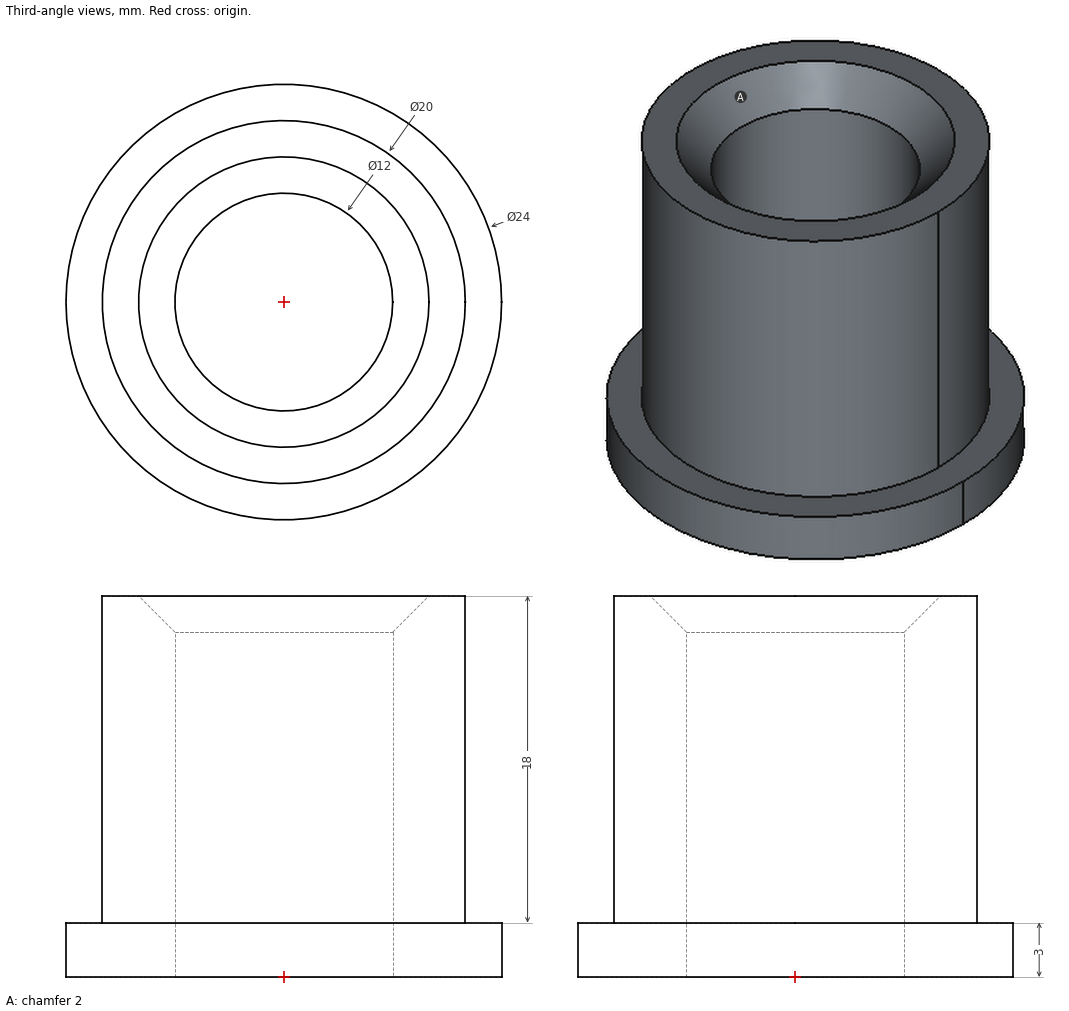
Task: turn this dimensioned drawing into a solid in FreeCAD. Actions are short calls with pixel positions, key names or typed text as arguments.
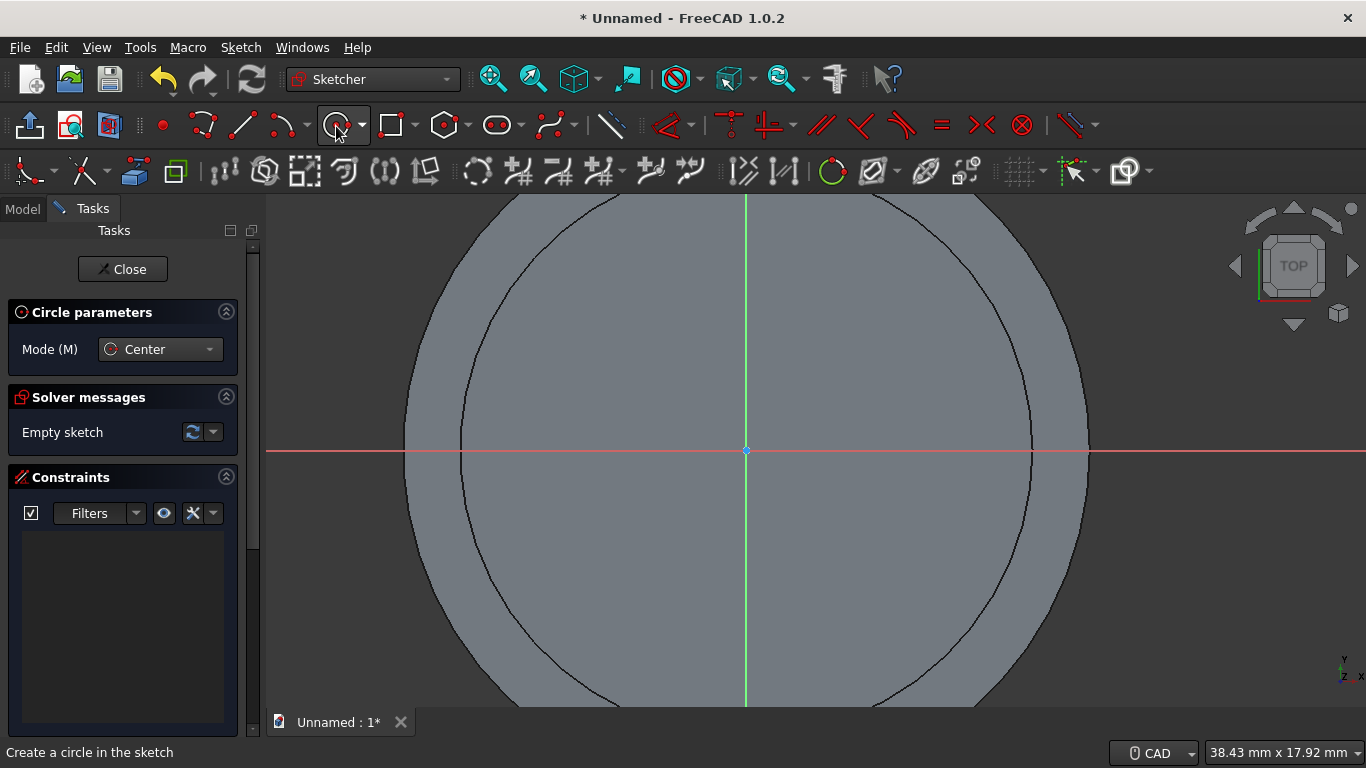
click(746, 450)
move(868, 329)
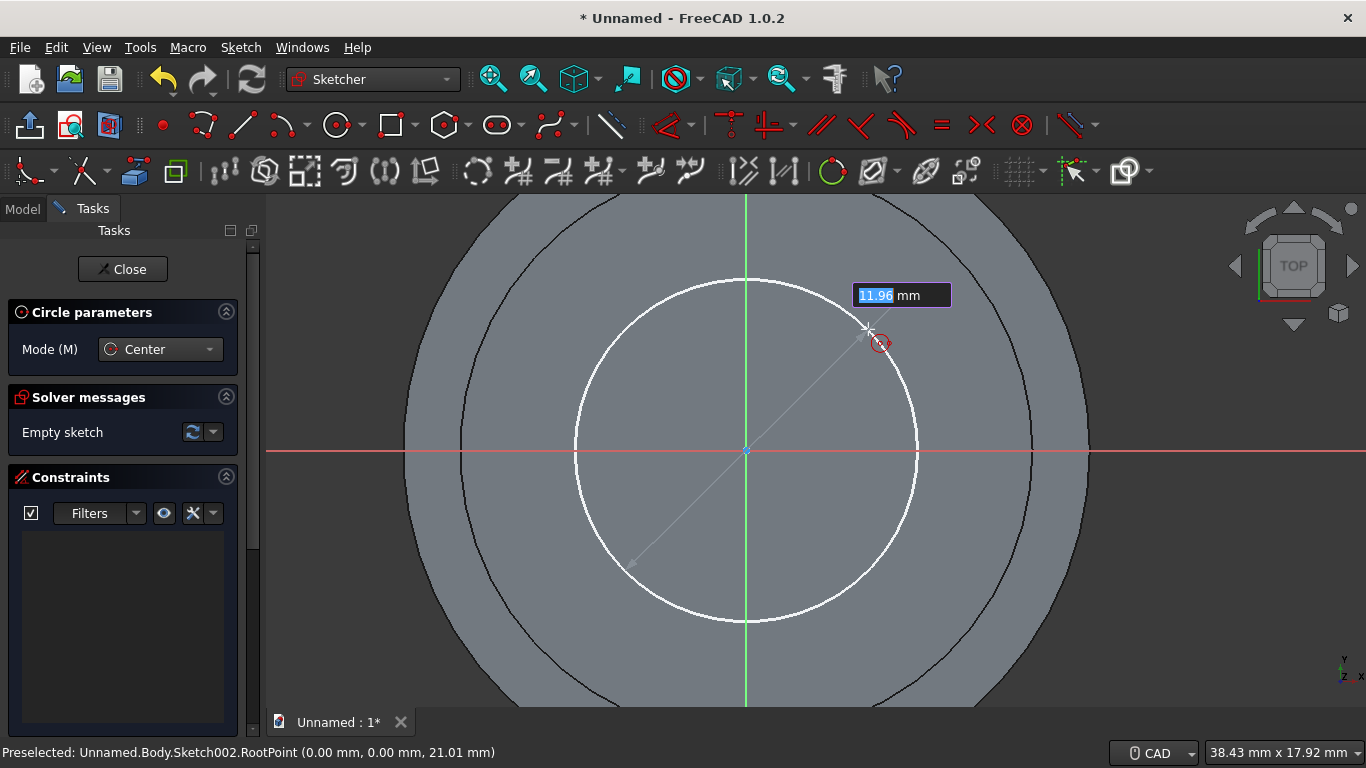
text(12)
key(Return)
key(Escape)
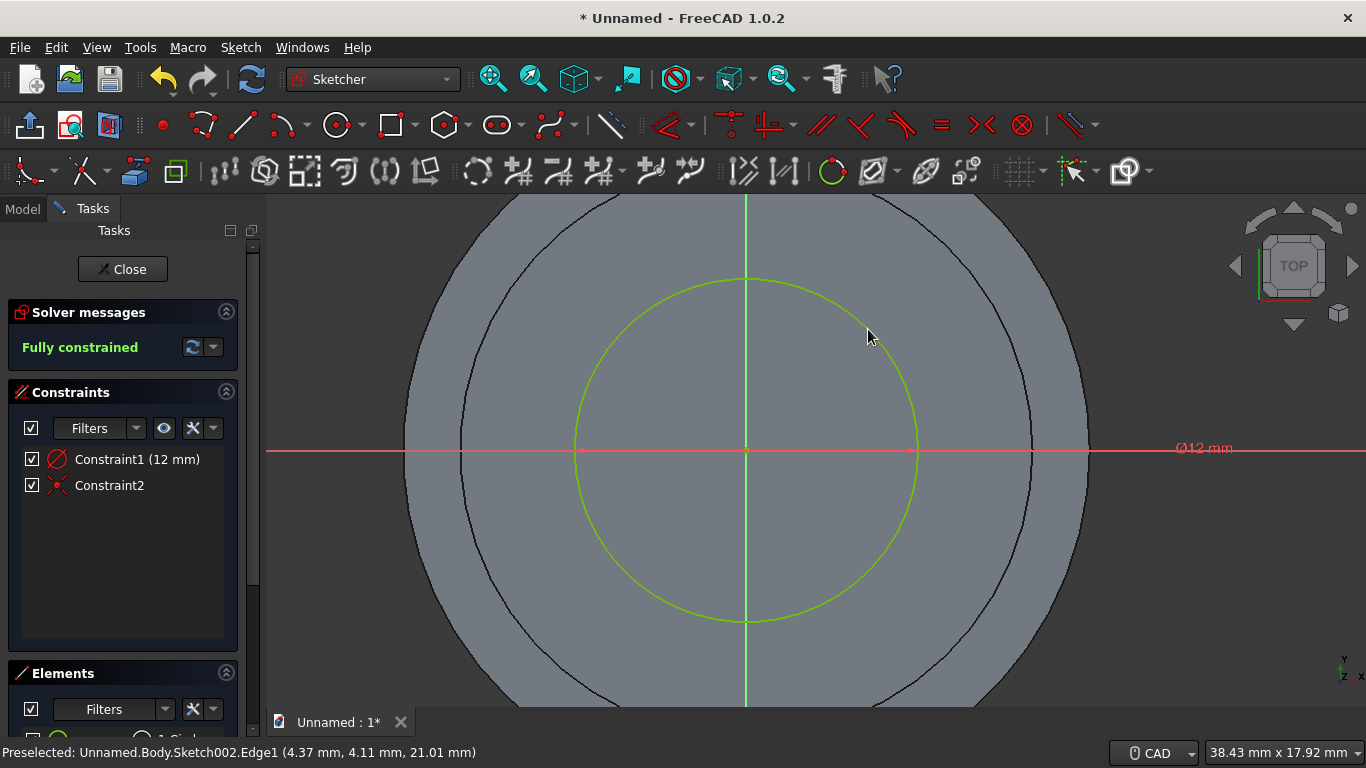
click(123, 269)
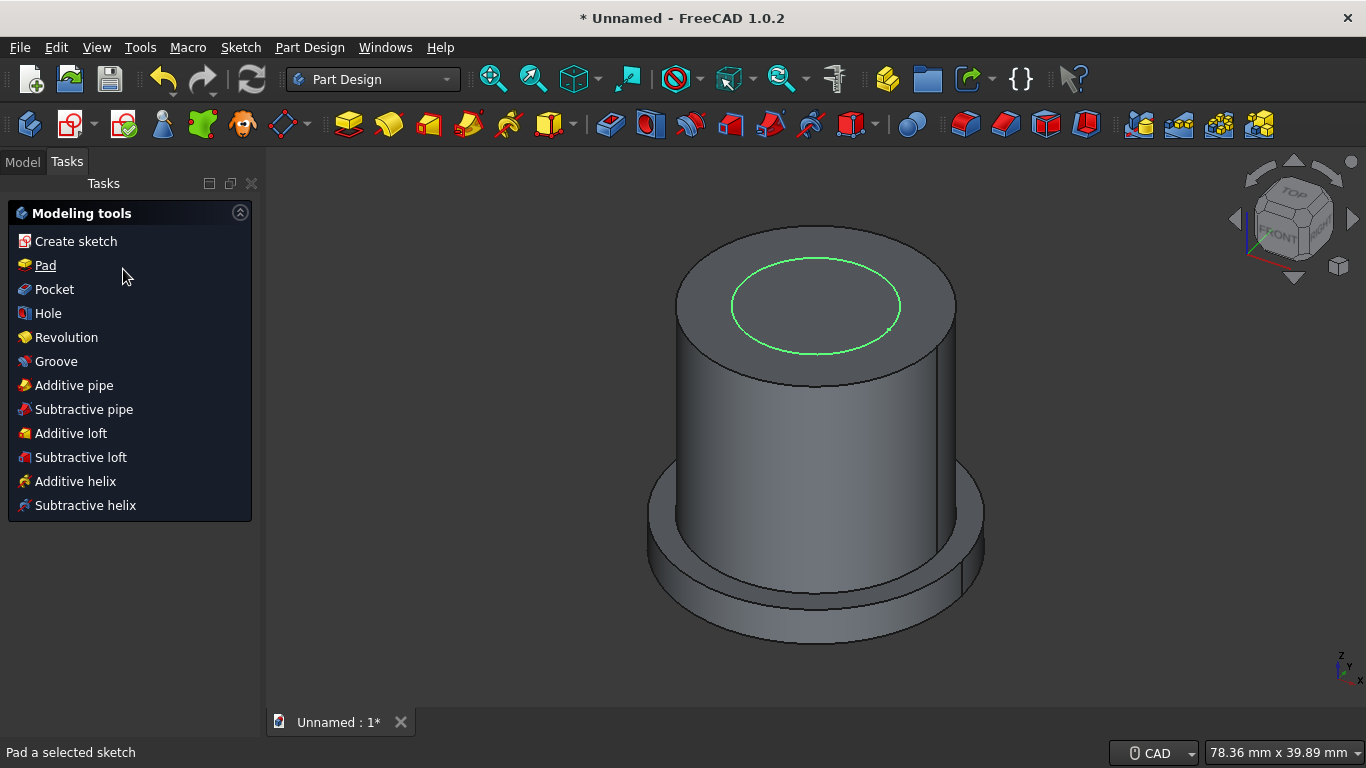
click(612, 124)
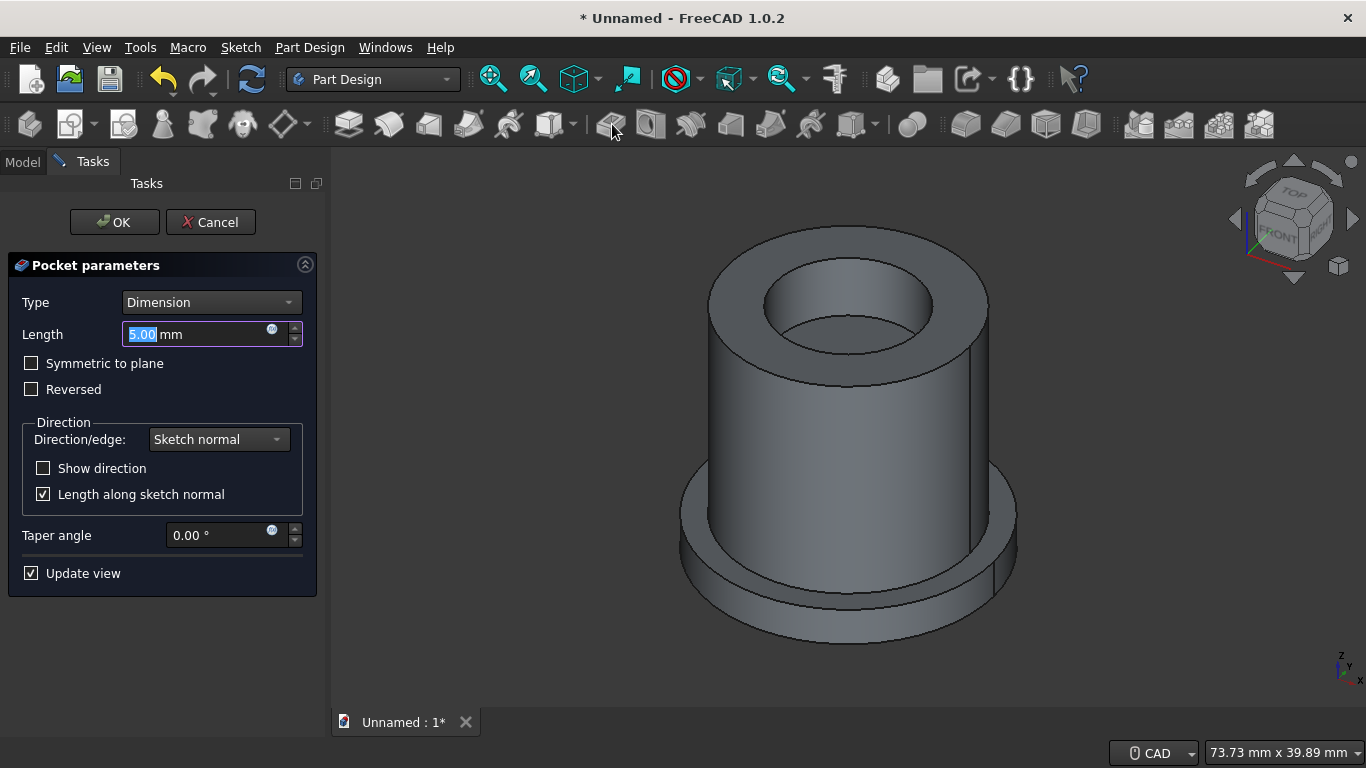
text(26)
key(Tab)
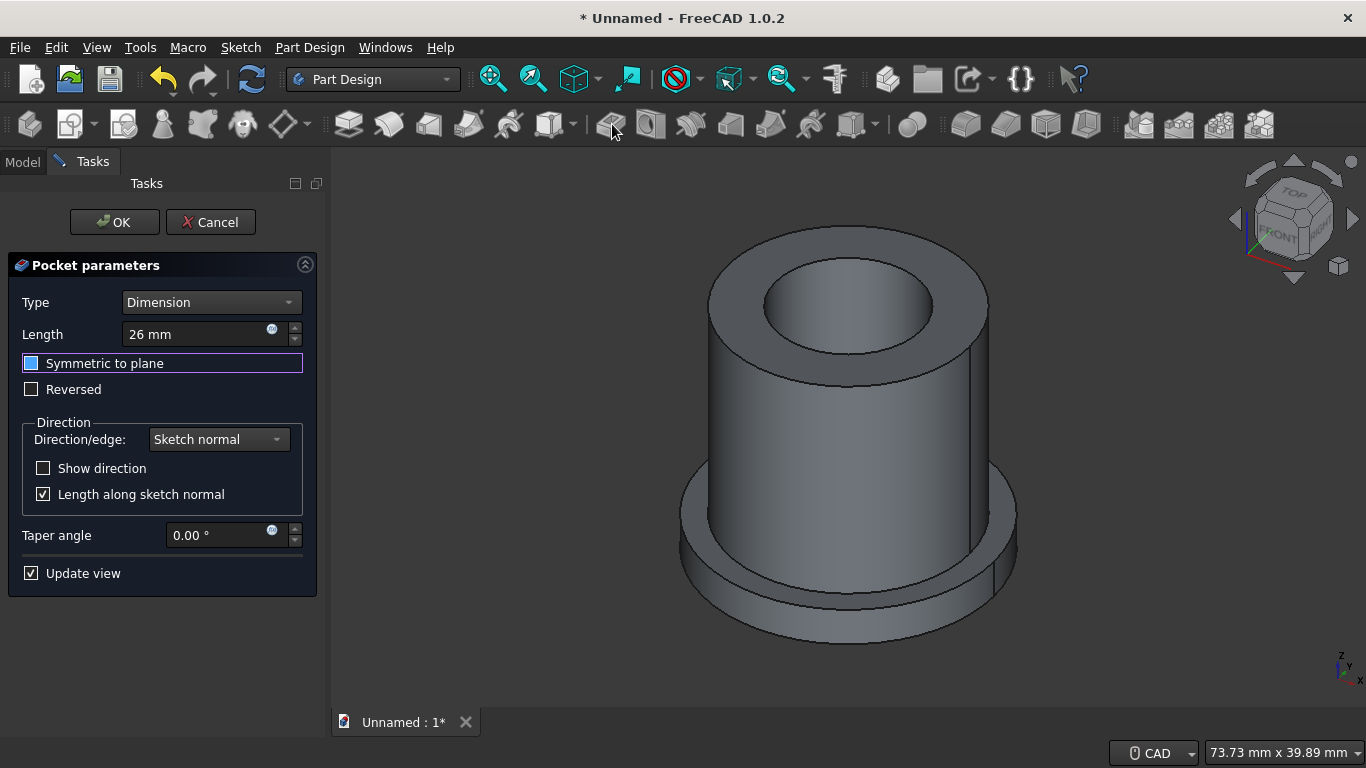
click(115, 222)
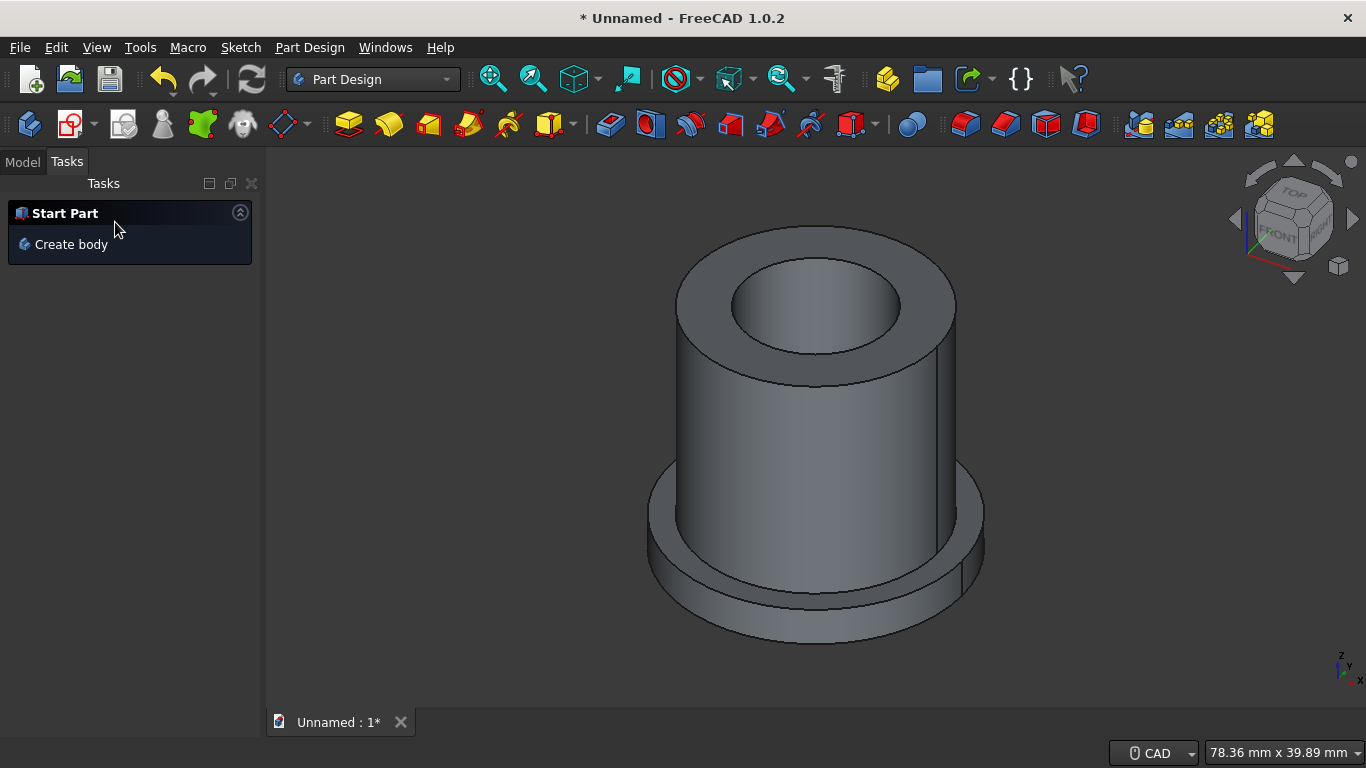
click(743, 281)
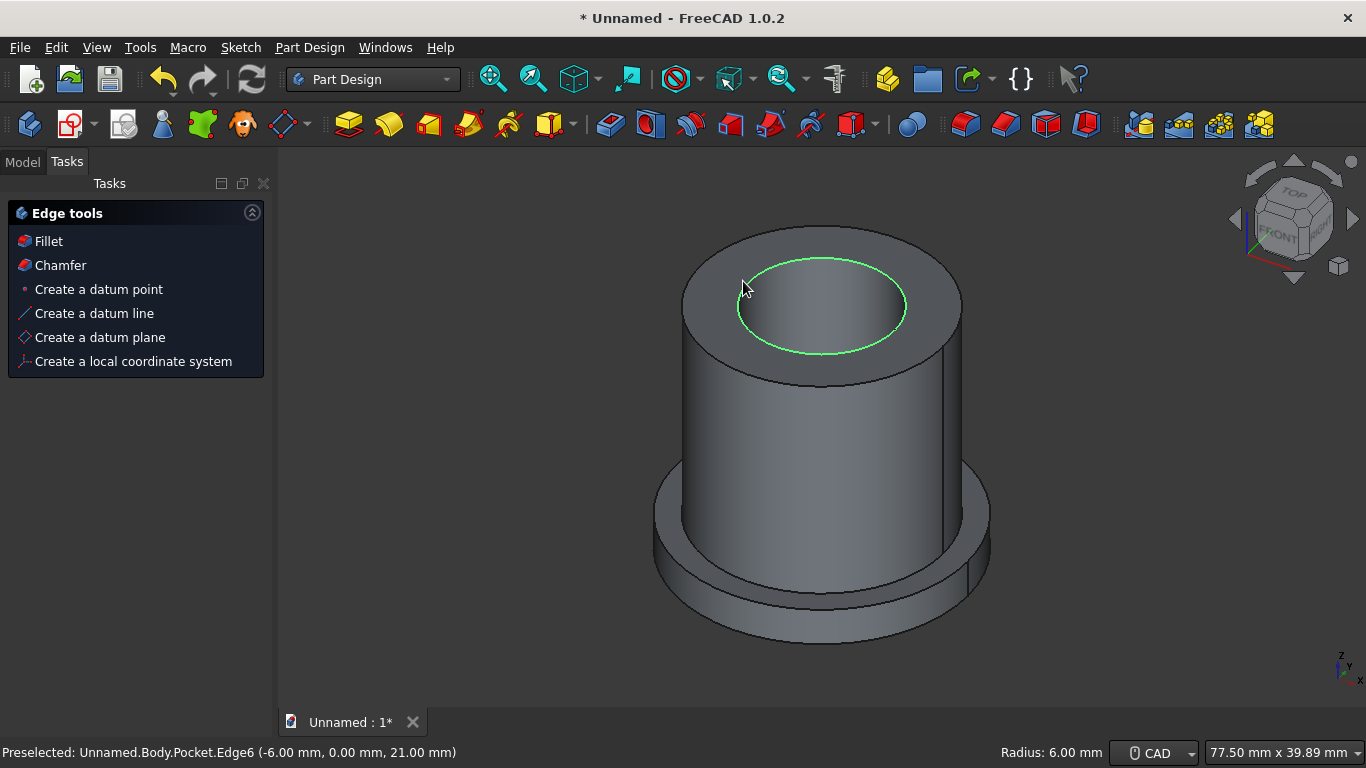
click(1006, 124)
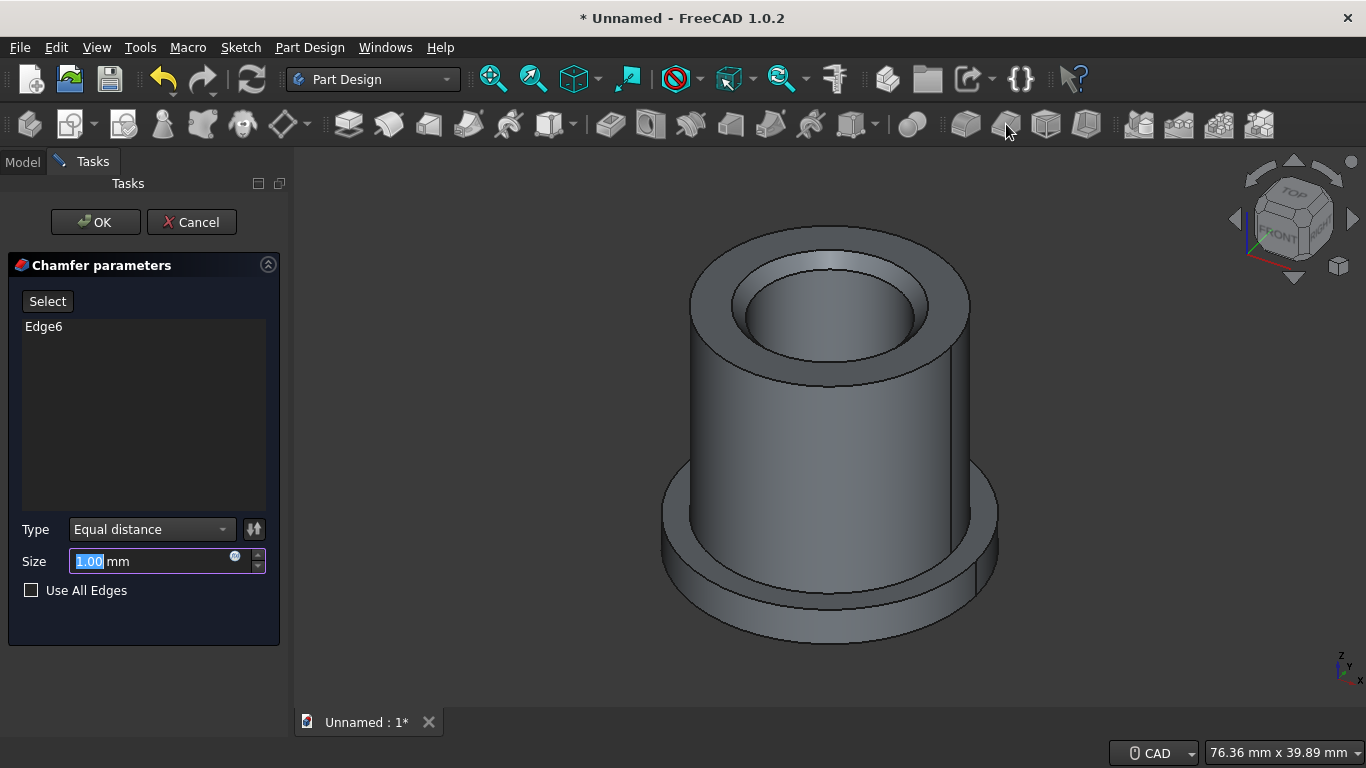
text(2)
key(Tab)